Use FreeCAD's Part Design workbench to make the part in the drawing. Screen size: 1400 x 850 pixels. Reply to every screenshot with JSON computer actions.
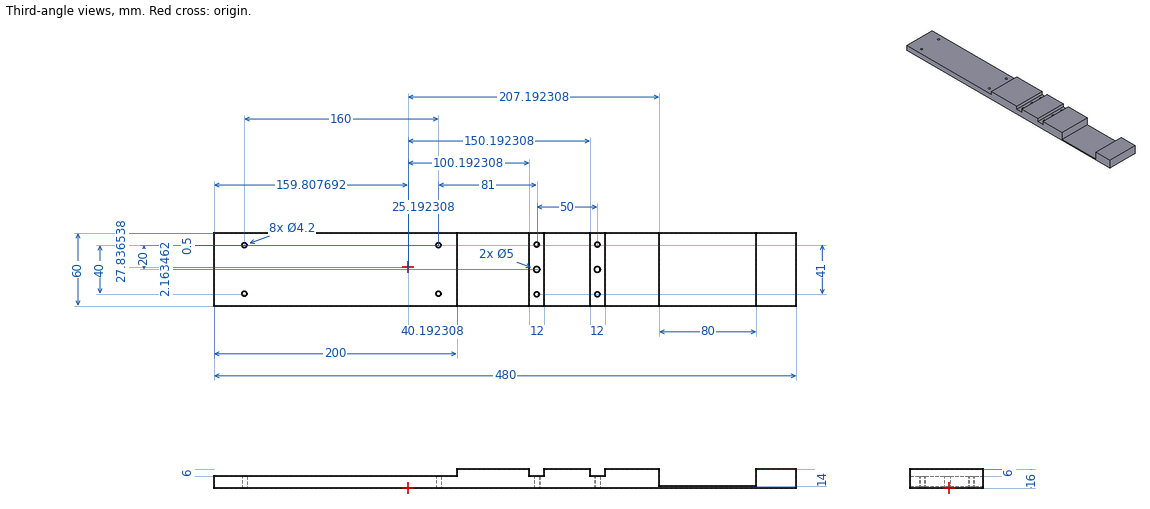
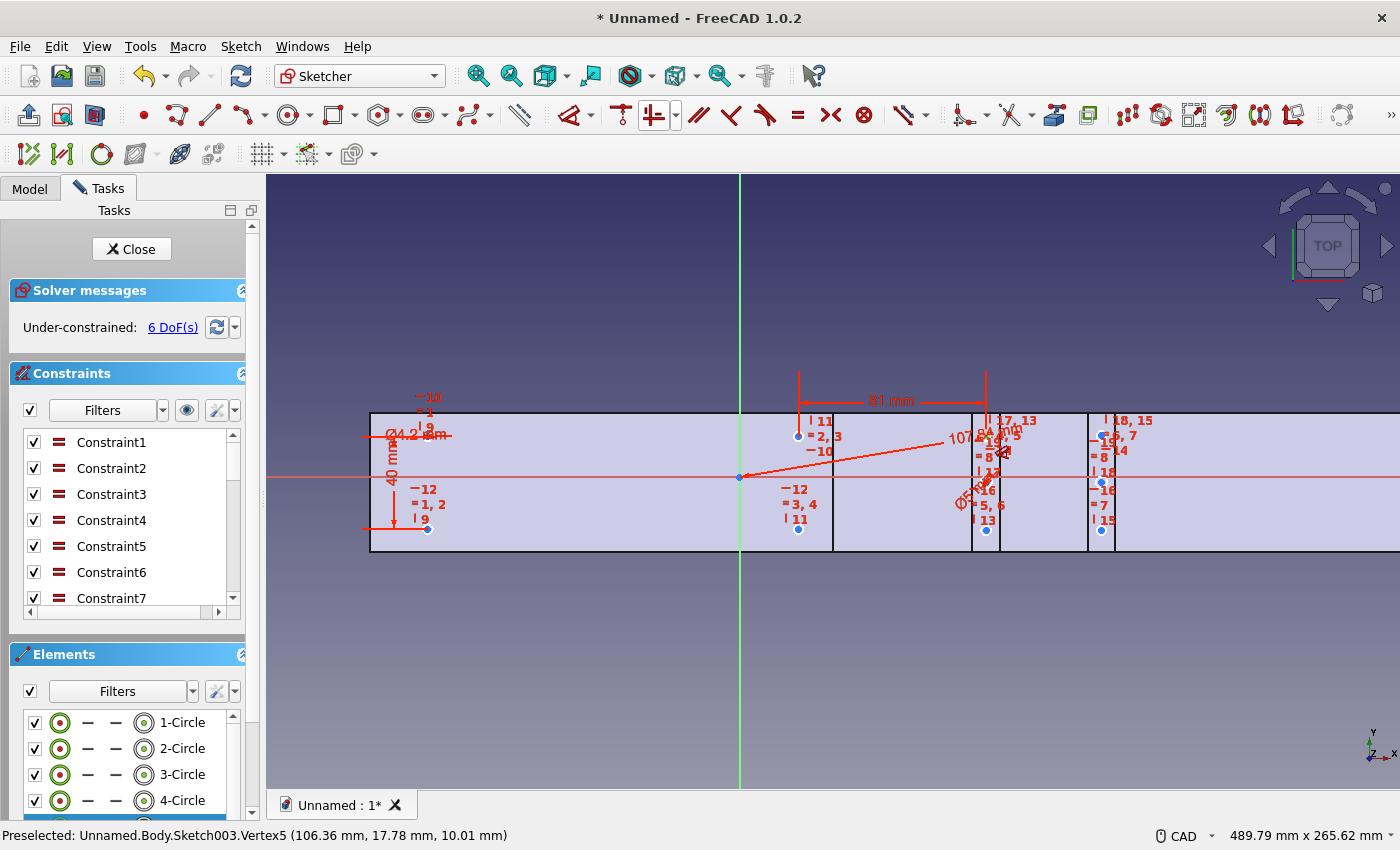
{"action": "left_click", "coordinate": [986, 530]}
{"action": "left_click", "coordinate": [1020, 461]}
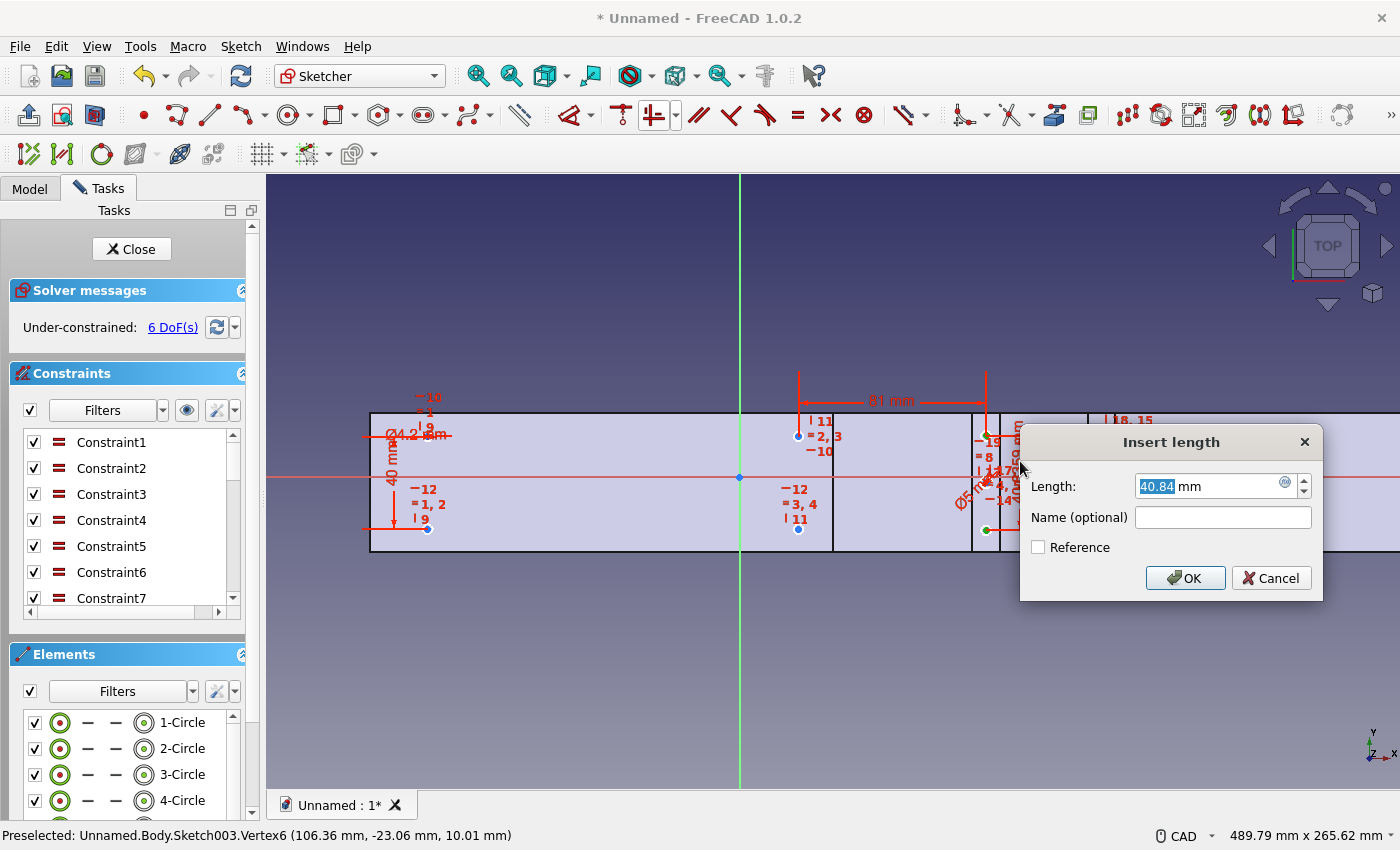
{"action": "type", "text": "41"}
{"action": "key", "text": "Return"}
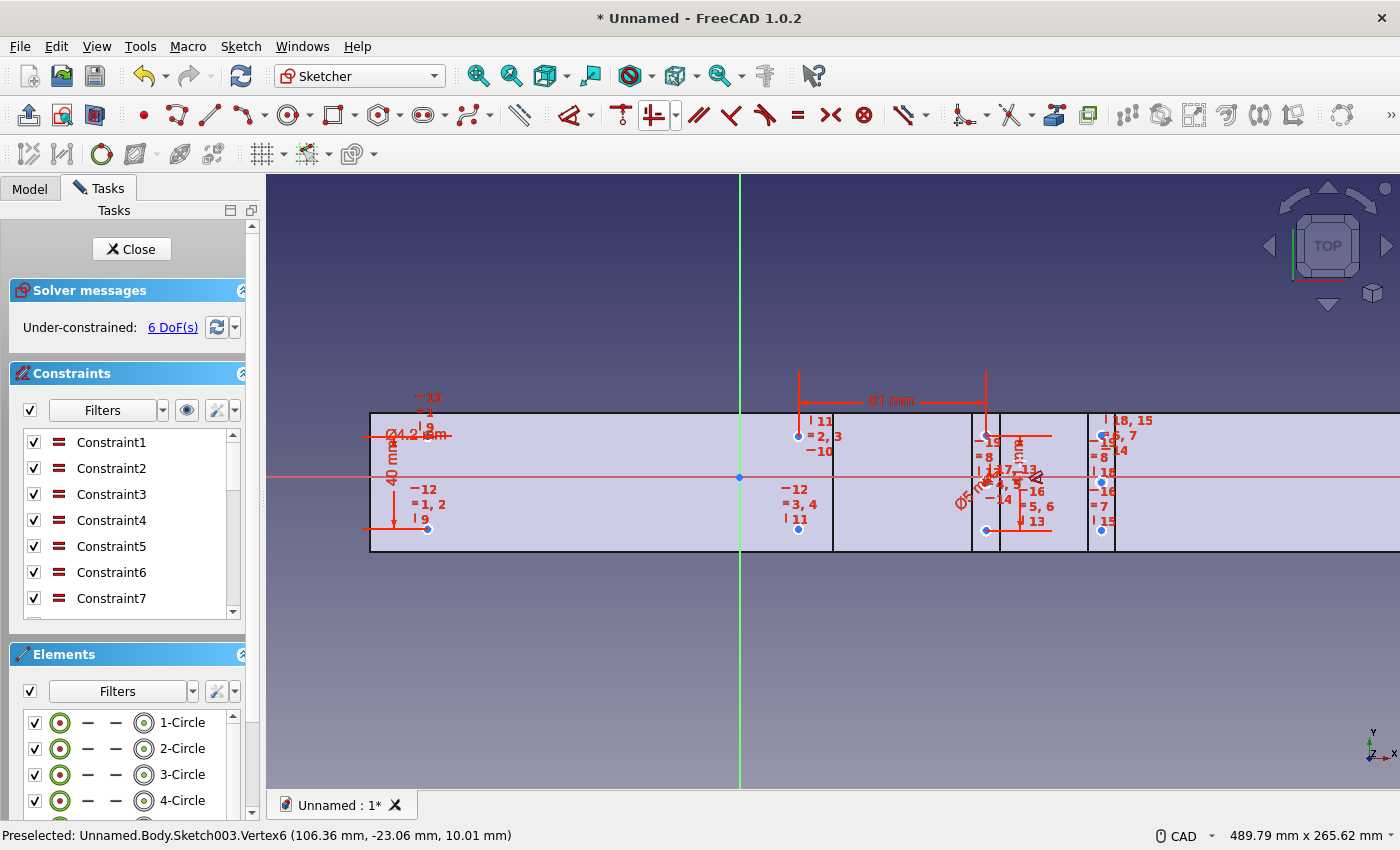
{"action": "left_click", "coordinate": [986, 436]}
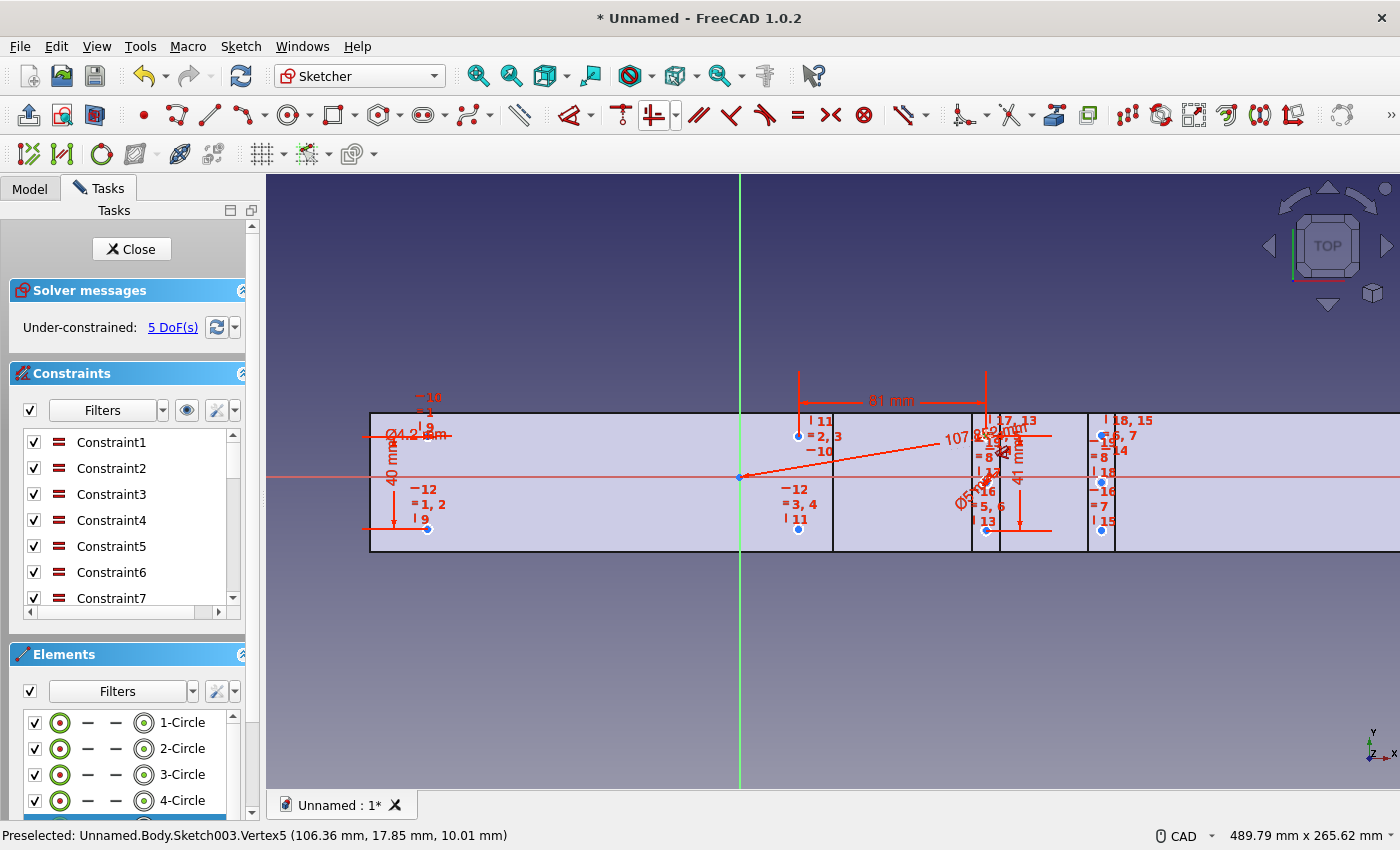
{"action": "left_click", "coordinate": [1102, 436]}
{"action": "left_click", "coordinate": [1044, 402]}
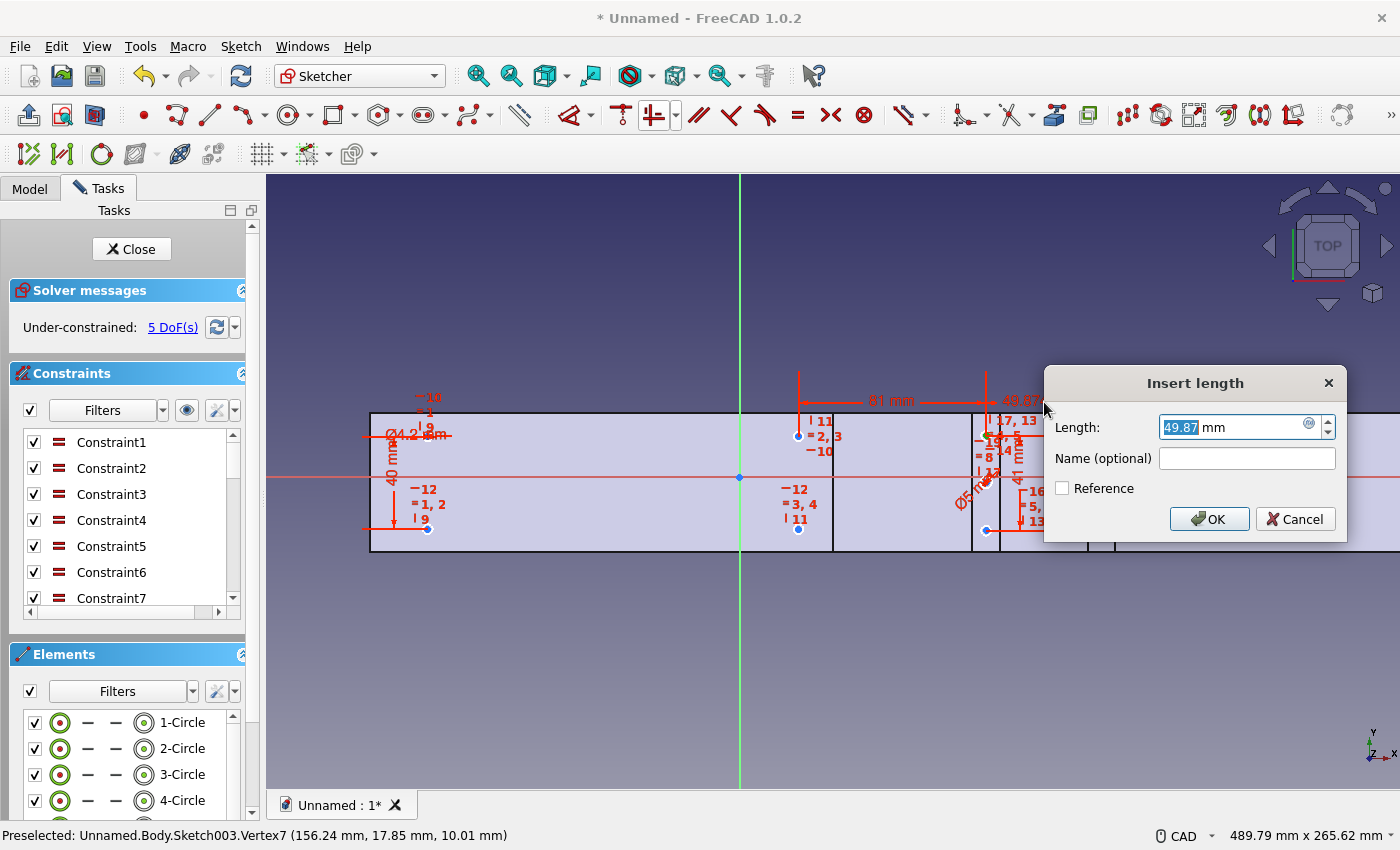
{"action": "type", "text": "50"}
{"action": "key", "text": "Return"}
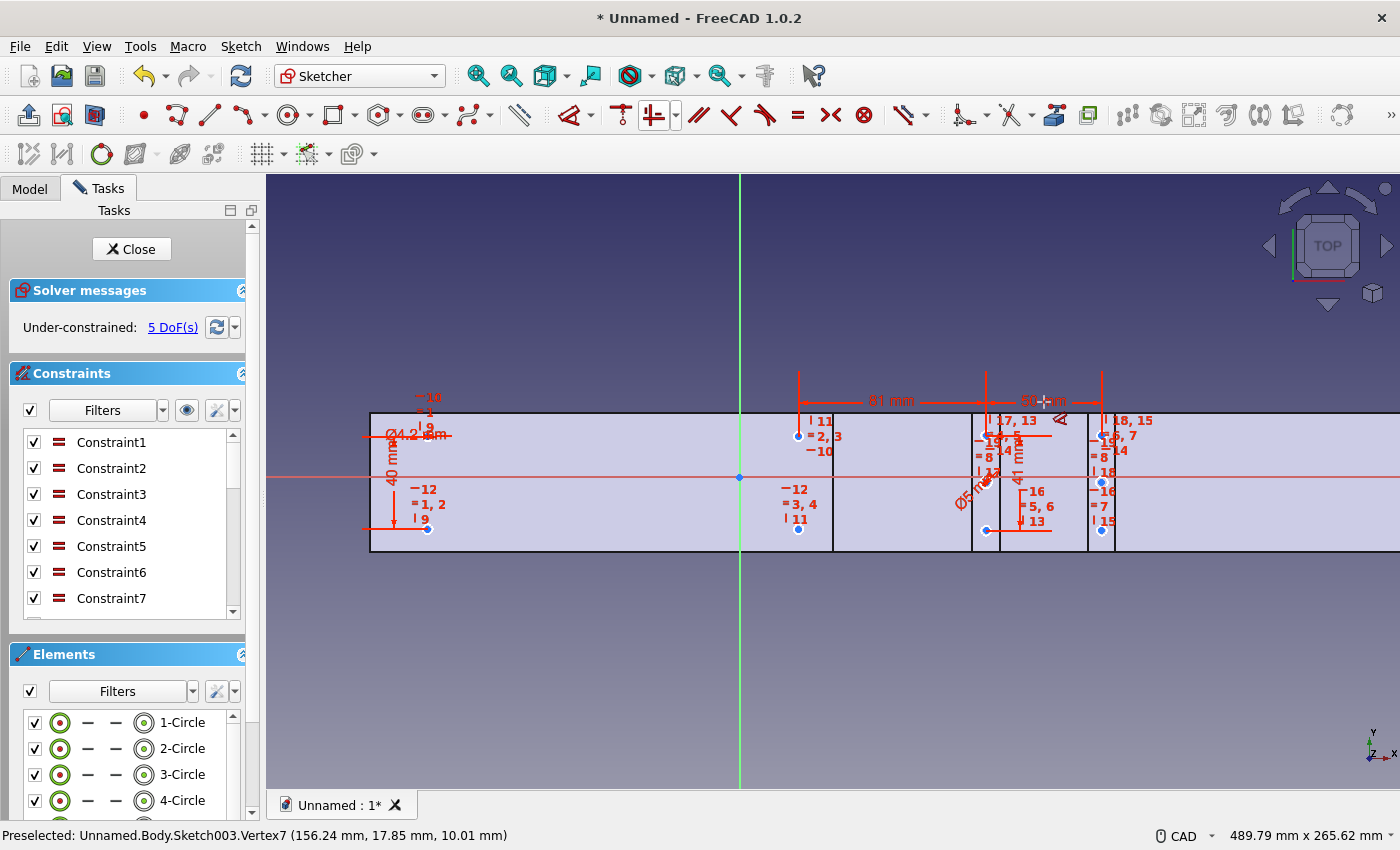
{"action": "left_click", "coordinate": [799, 437]}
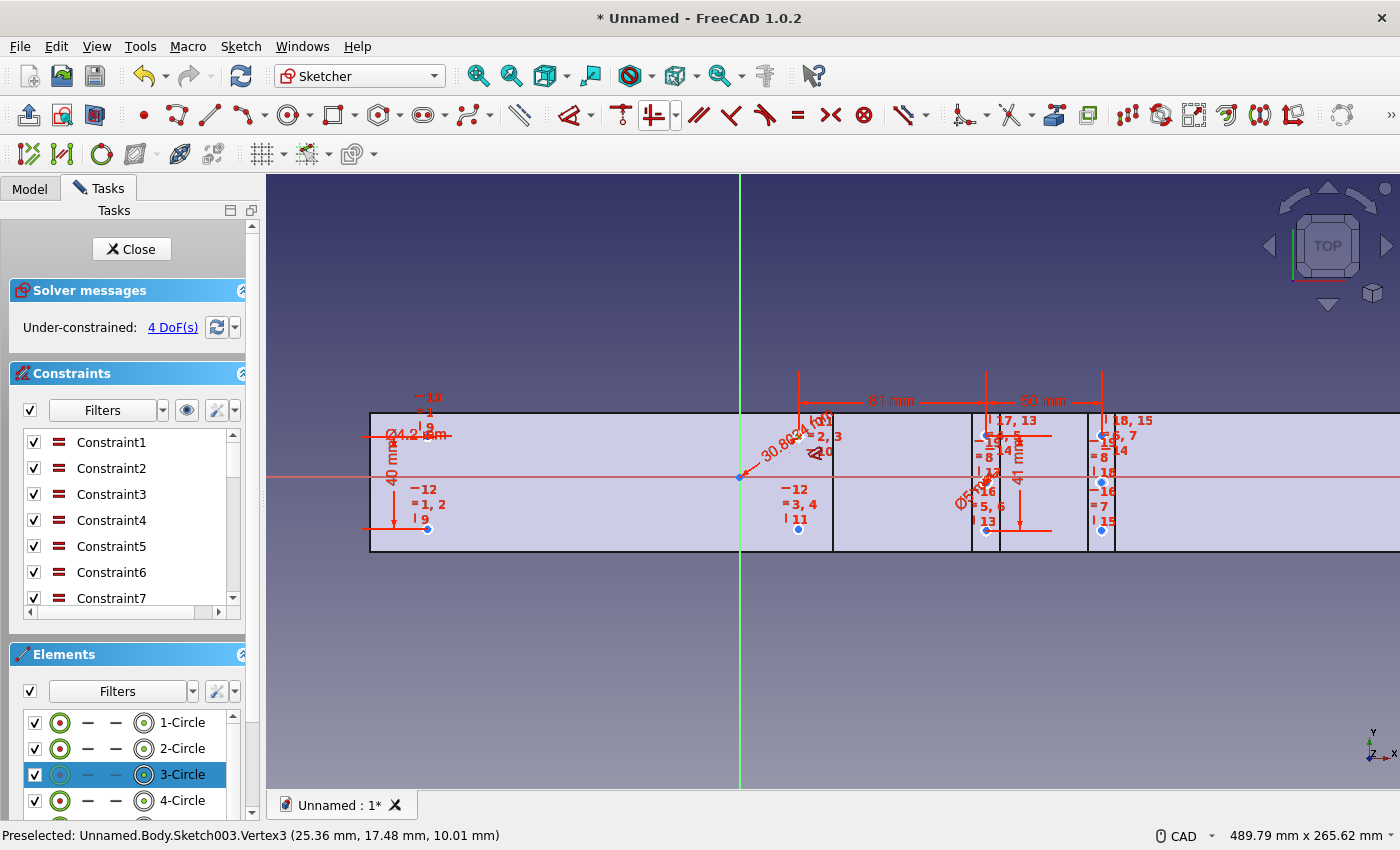
{"action": "left_click", "coordinate": [986, 482]}
{"action": "left_click", "coordinate": [765, 460]}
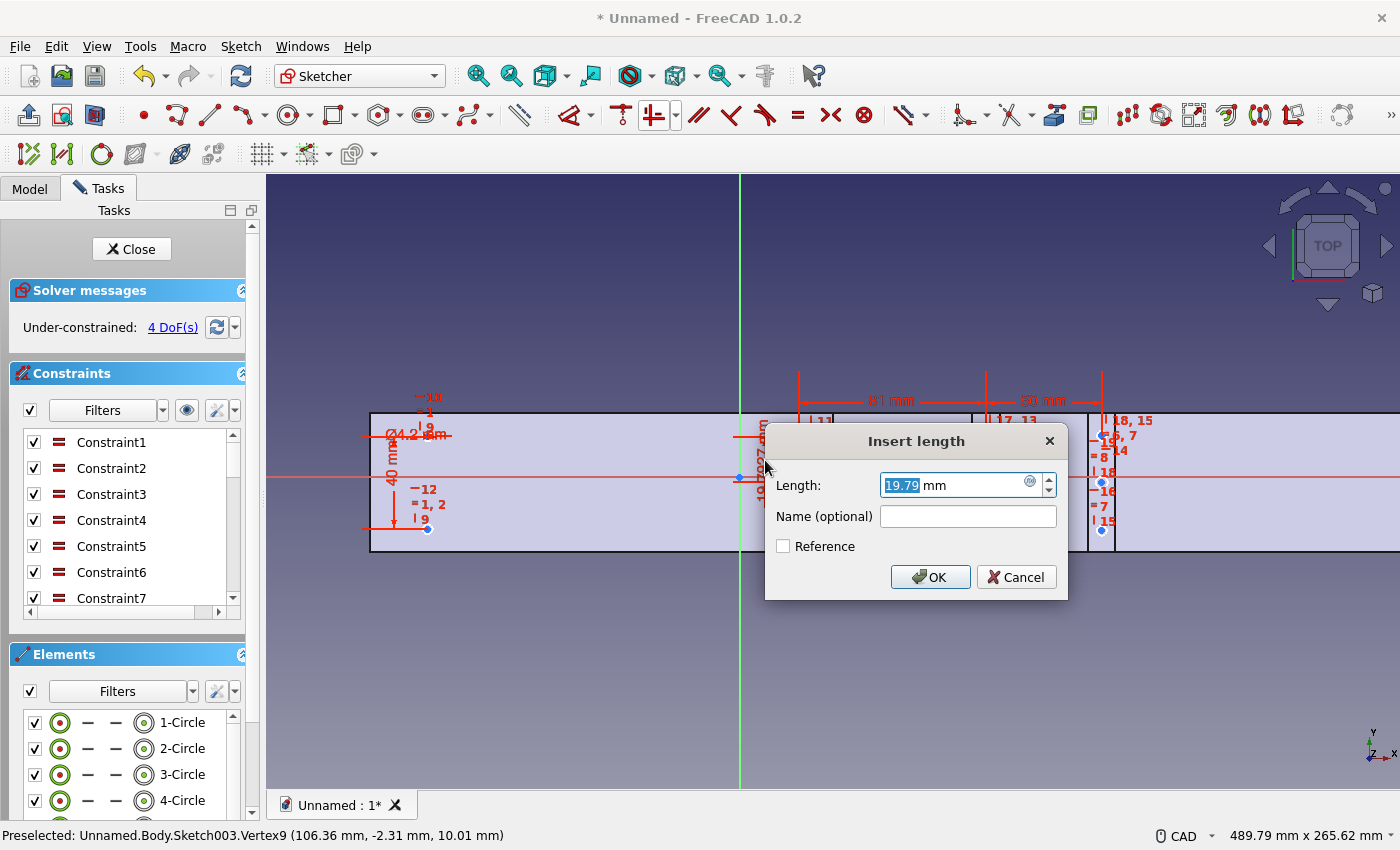
{"action": "type", "text": "20"}
{"action": "key", "text": "Return"}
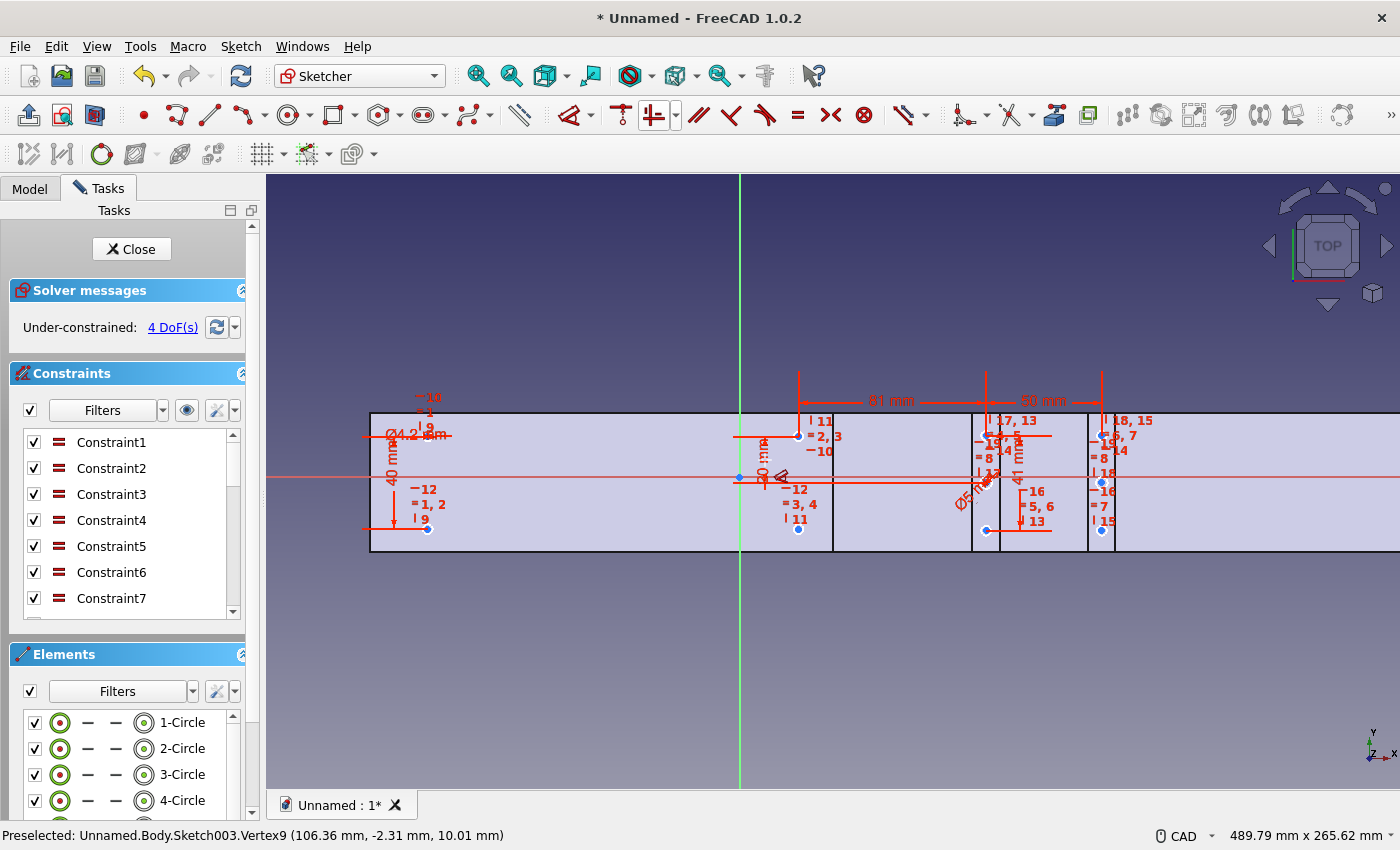
{"action": "left_click", "coordinate": [428, 437]}